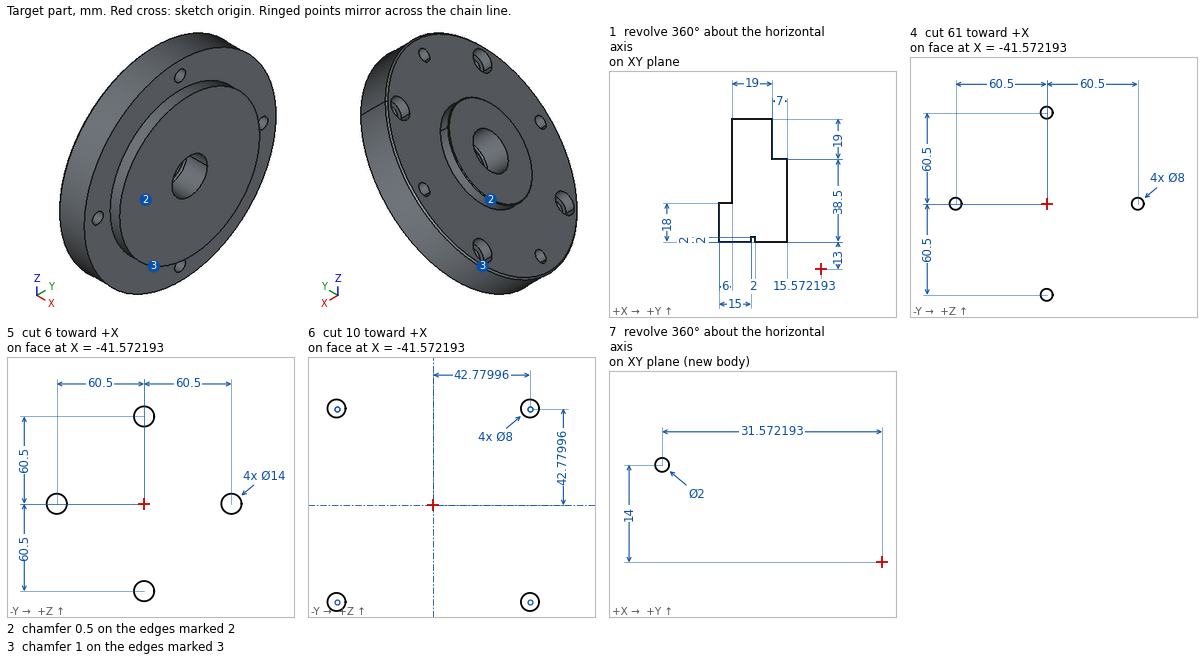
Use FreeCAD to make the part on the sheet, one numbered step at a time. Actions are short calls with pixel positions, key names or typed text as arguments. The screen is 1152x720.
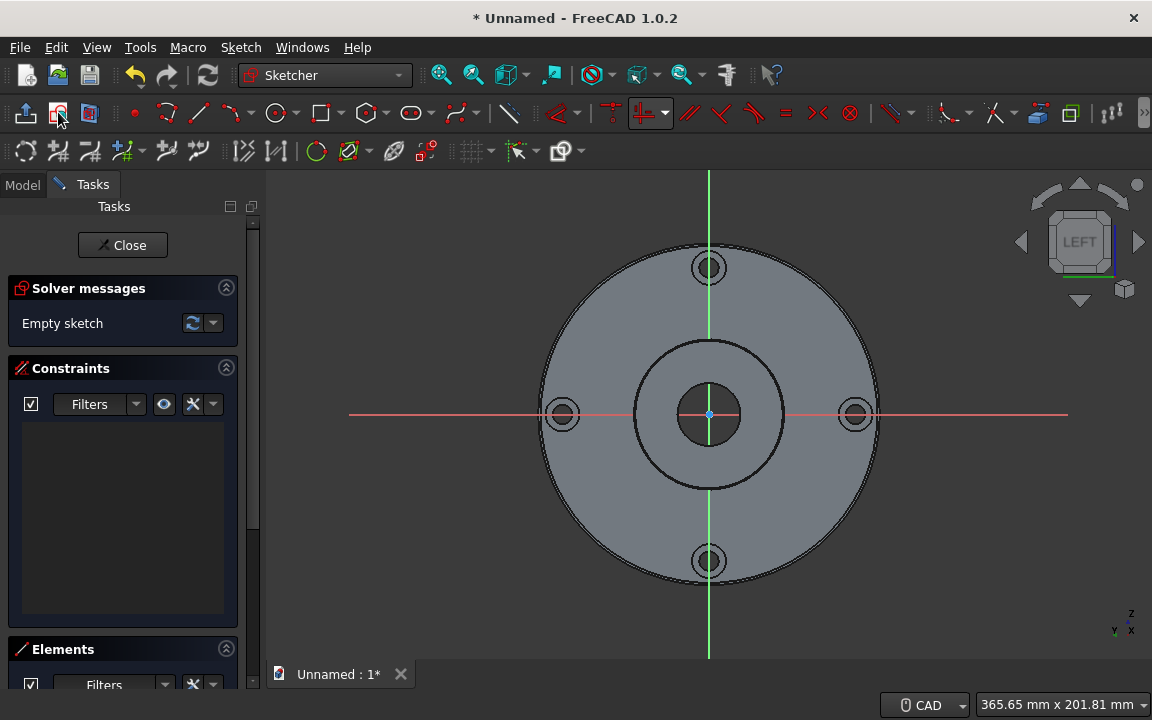
click(276, 114)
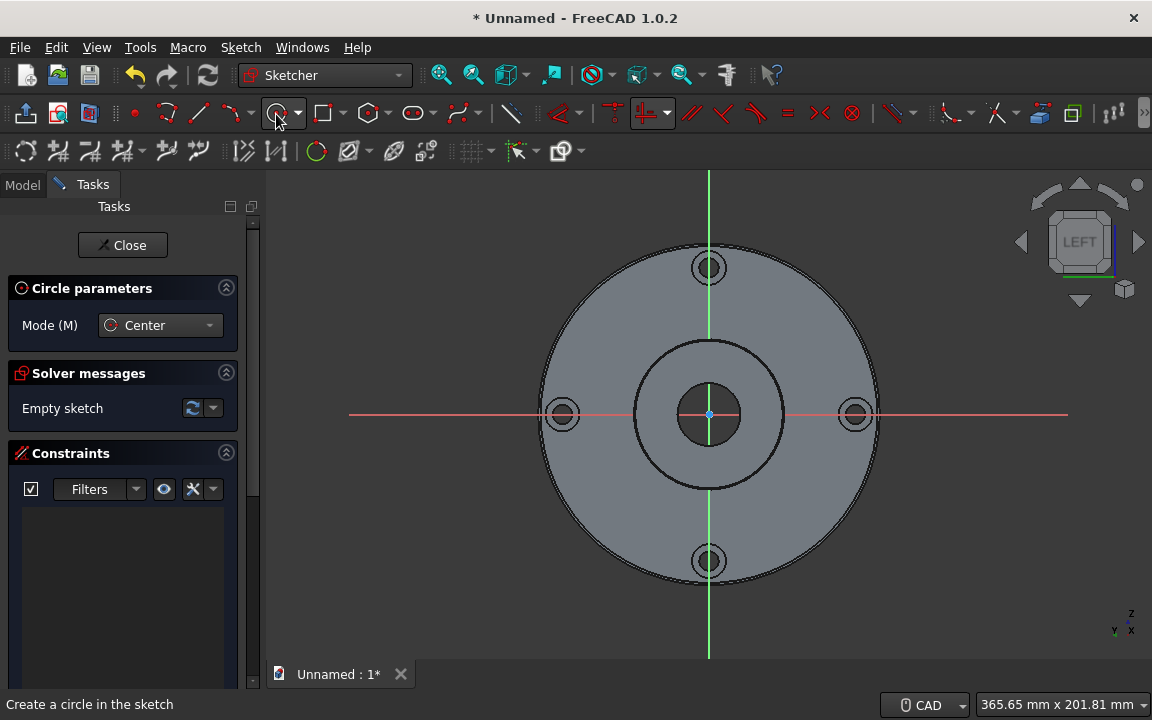
scroll(813, 311, up, 5)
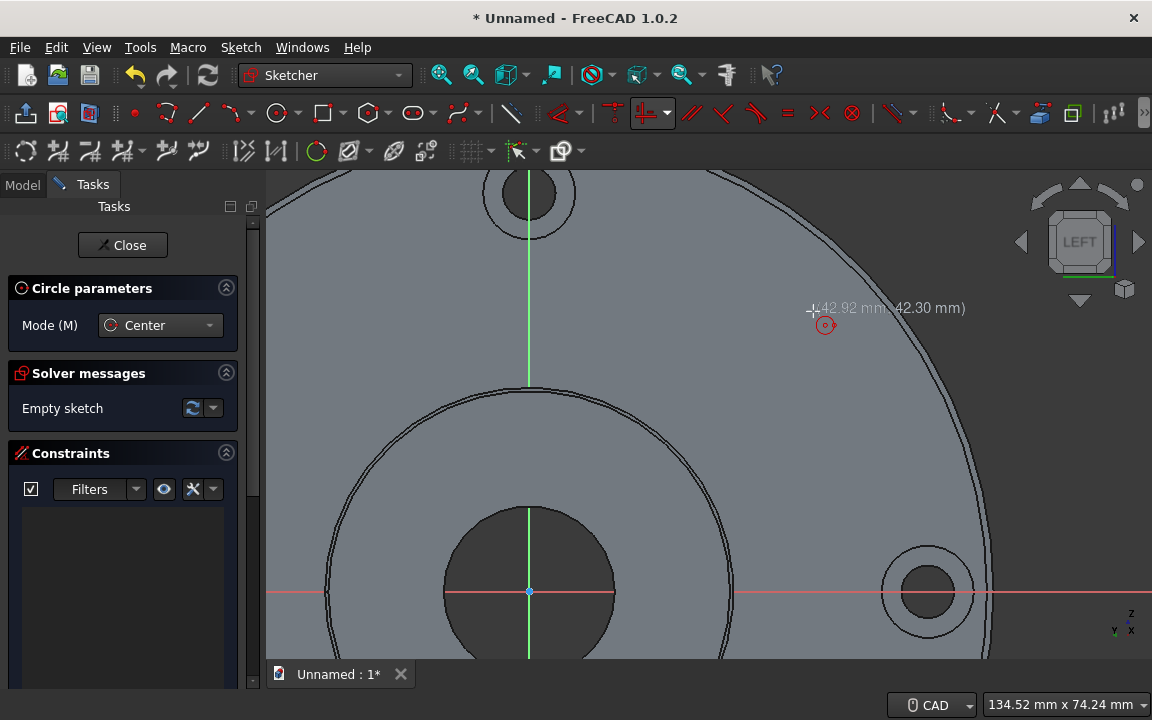
click(811, 310)
move(830, 291)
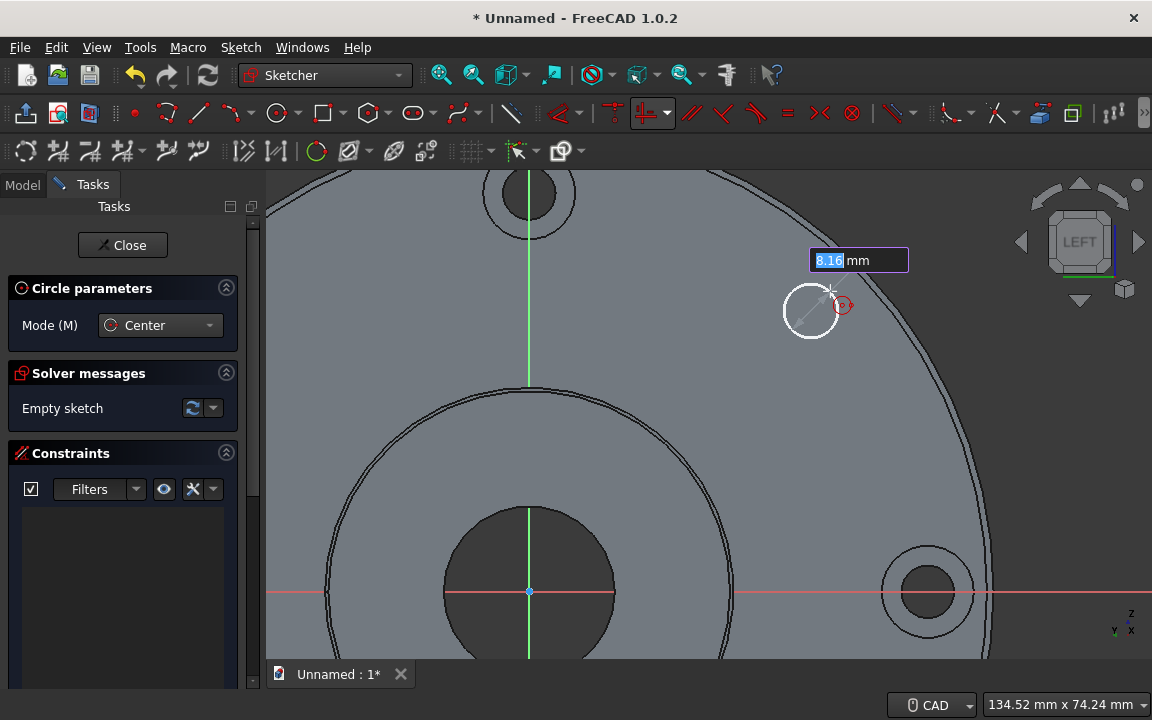
text(8)
key(Return)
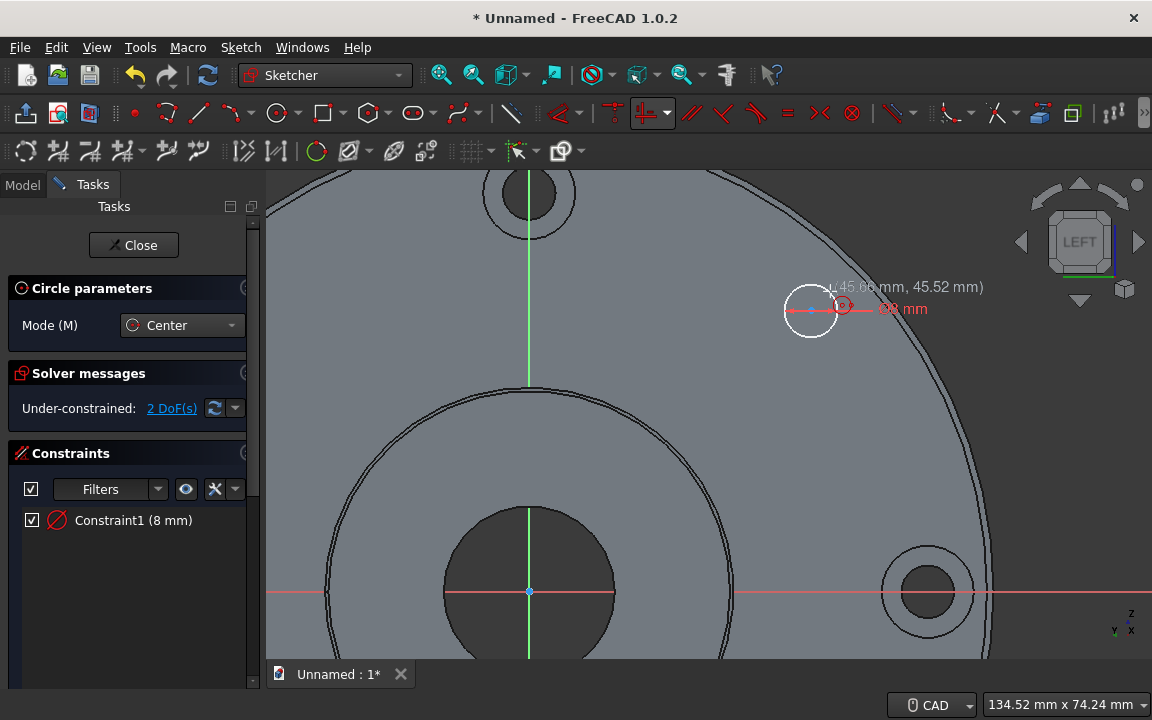
scroll(731, 270, down, 4)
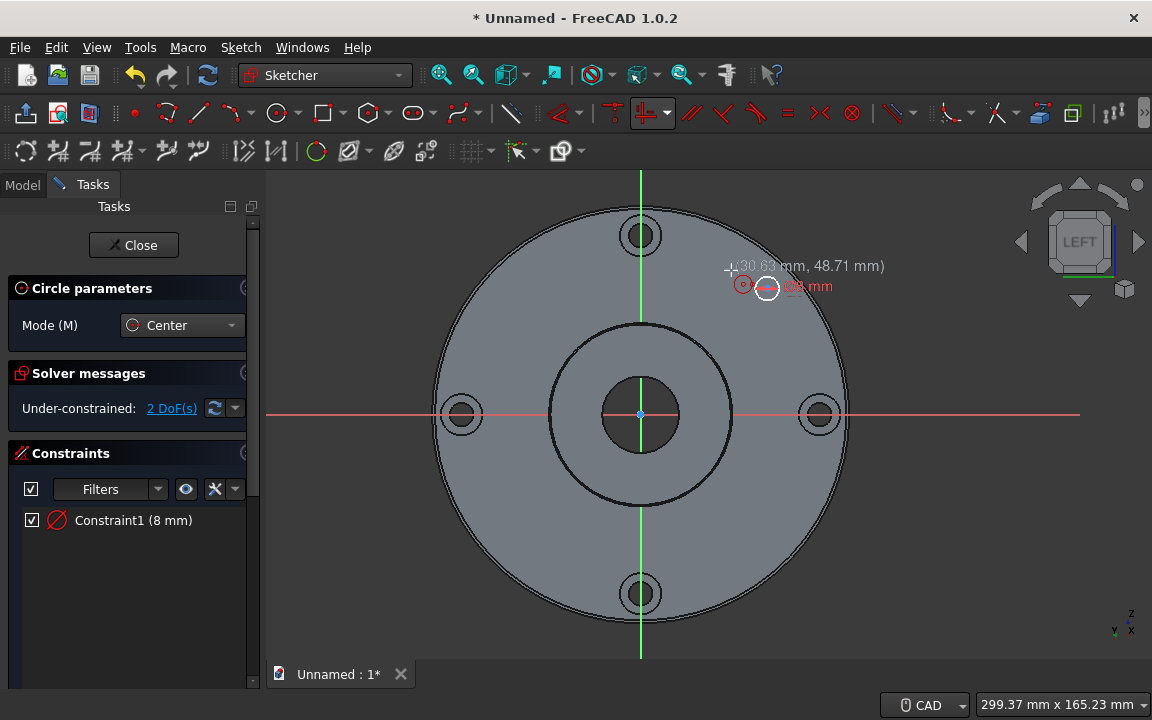
scroll(514, 288, up, 4)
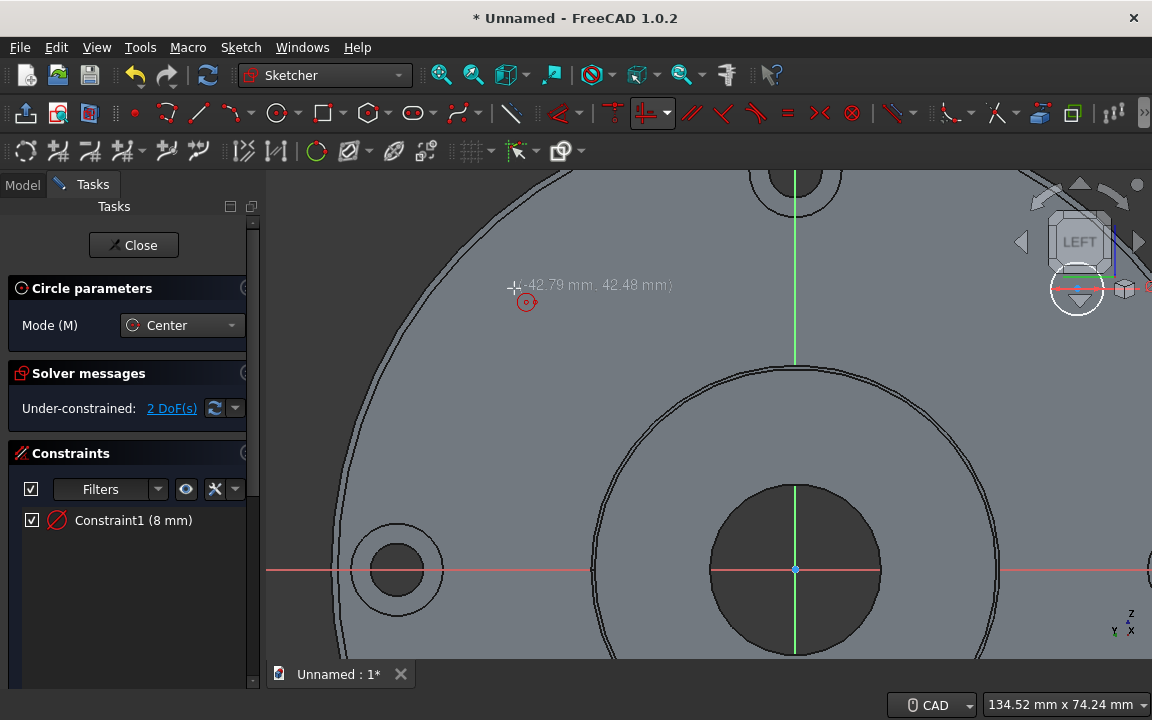
click(514, 288)
move(532, 269)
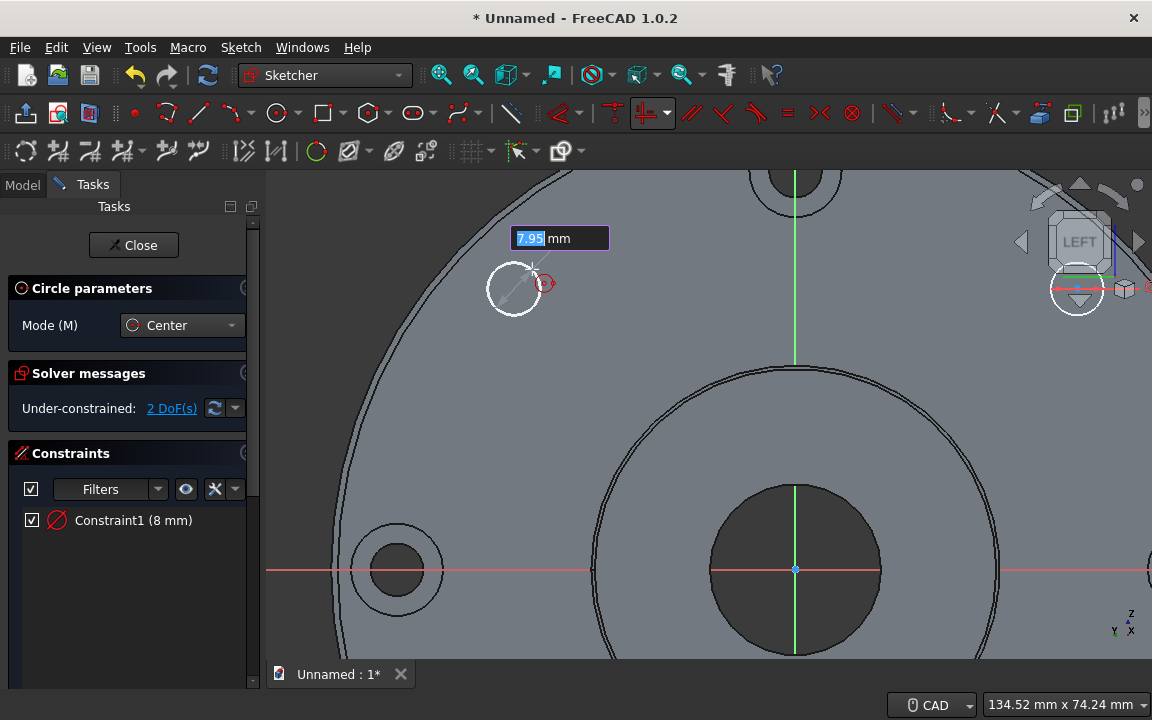
text(8)
key(Return)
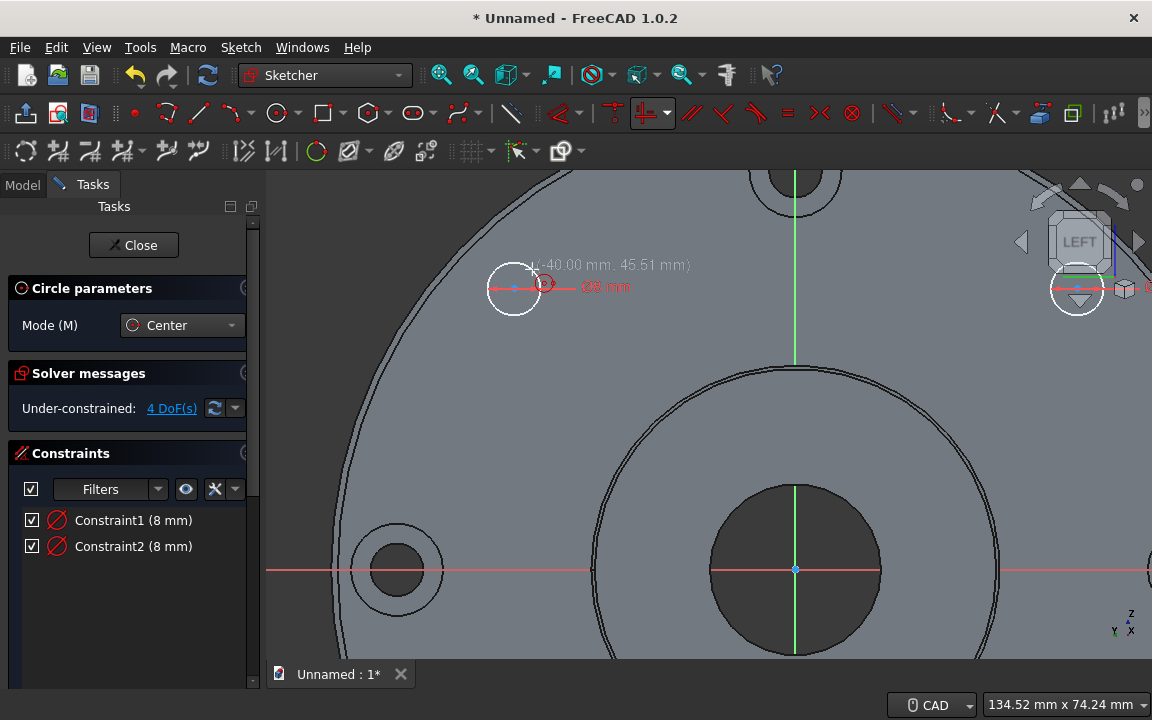
scroll(514, 288, down, 4)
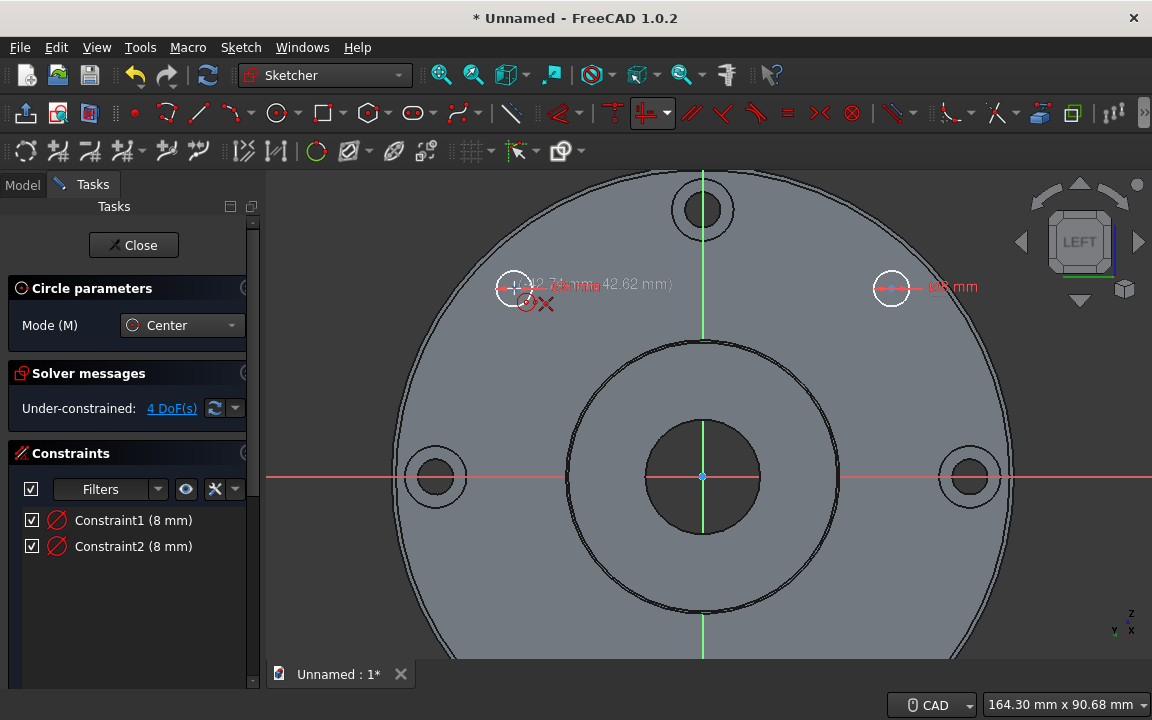
scroll(767, 541, up, 4)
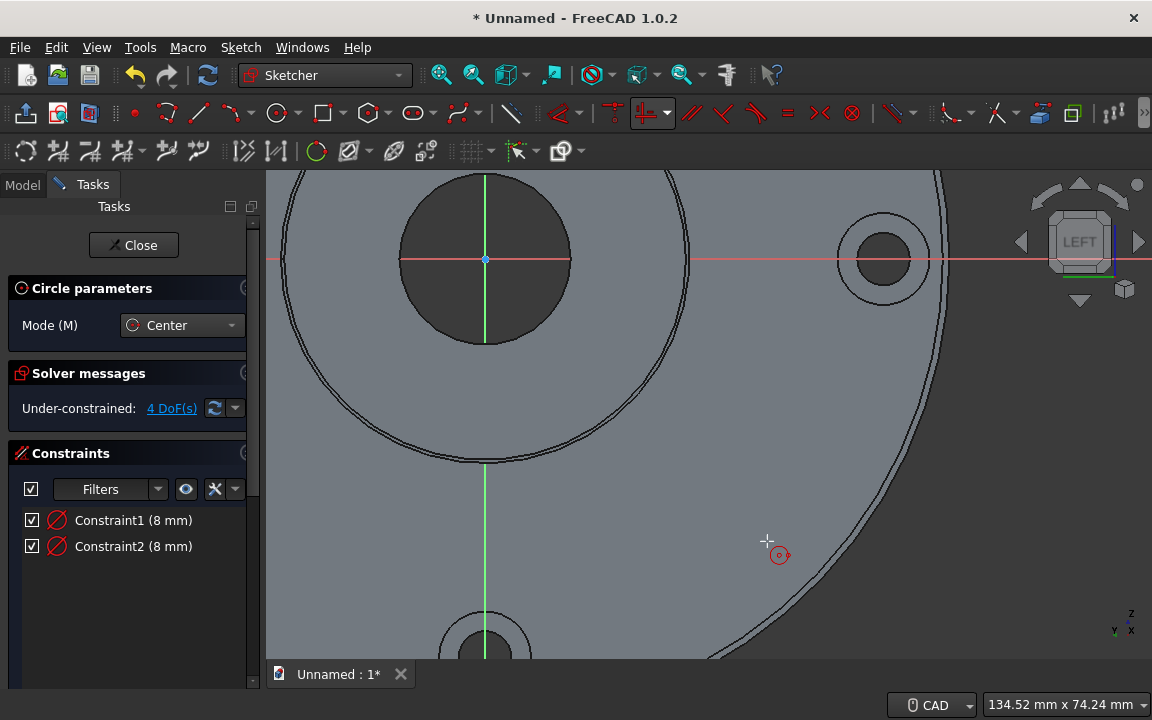
click(767, 541)
move(785, 522)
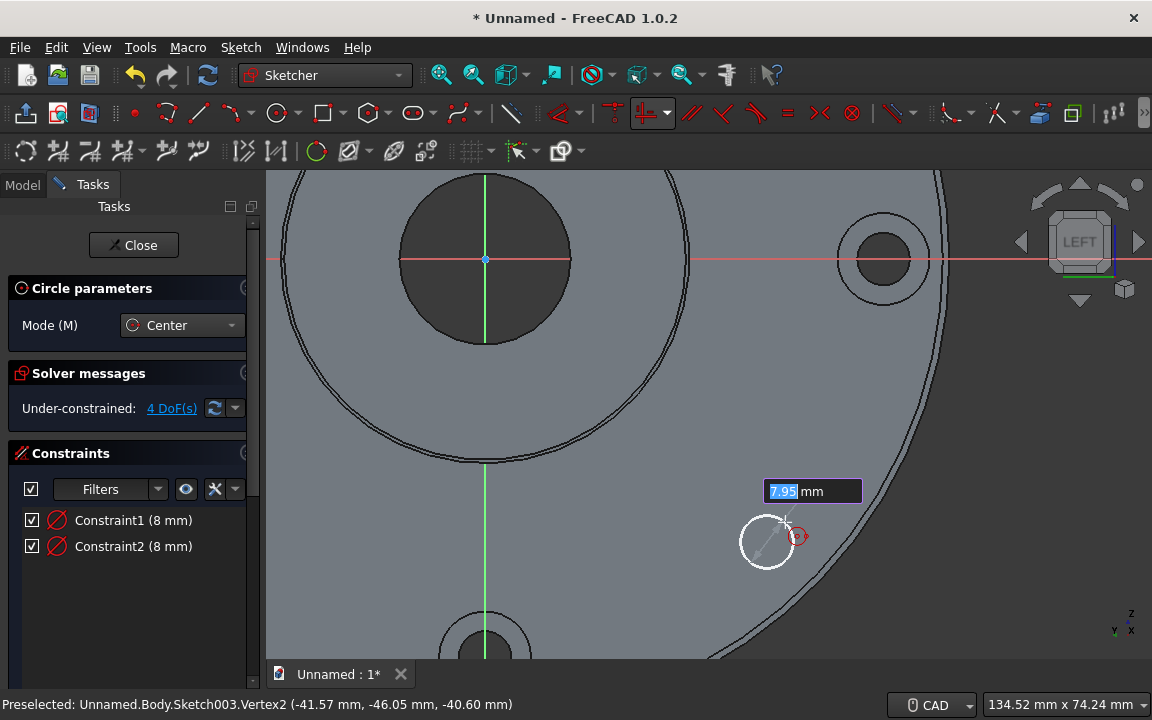
text(8)
key(Return)